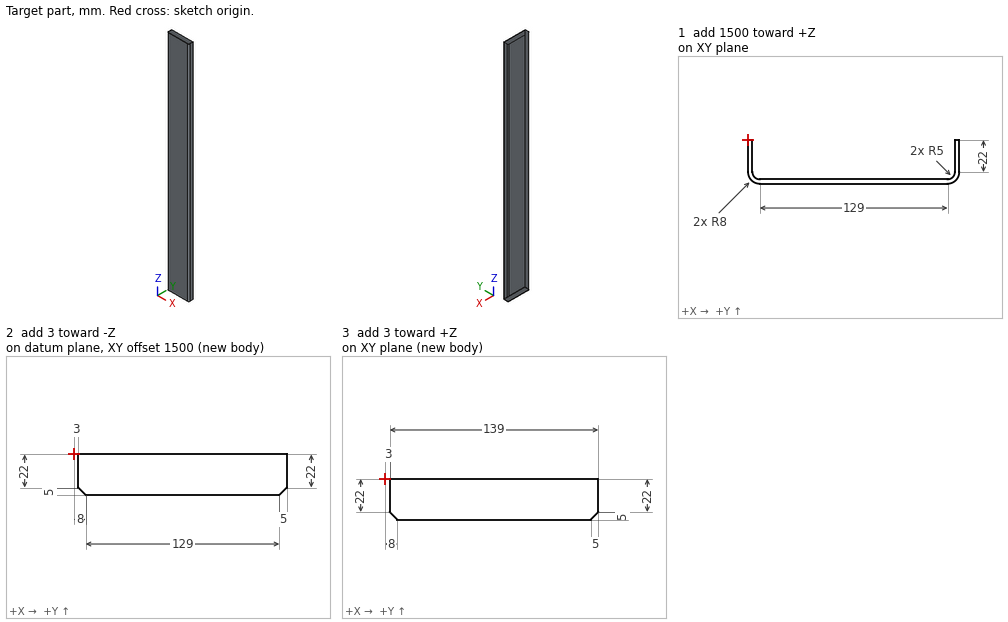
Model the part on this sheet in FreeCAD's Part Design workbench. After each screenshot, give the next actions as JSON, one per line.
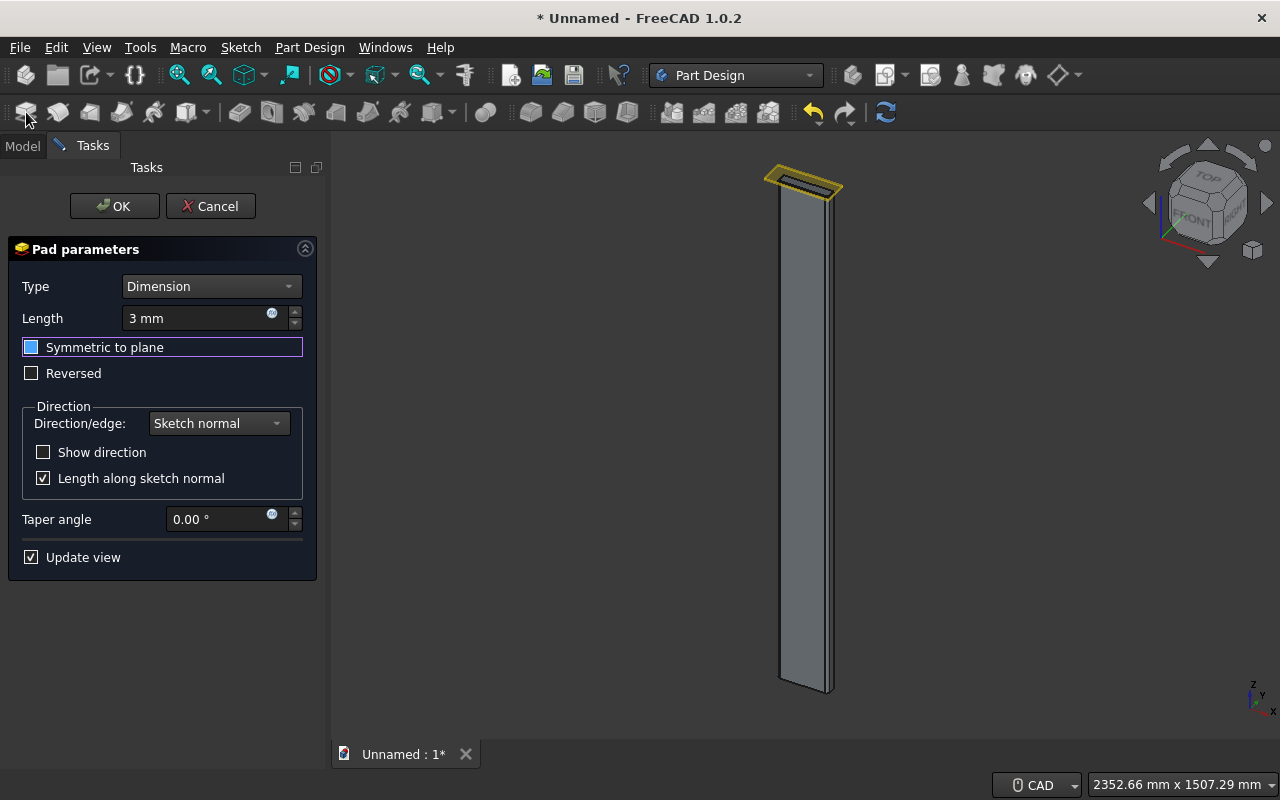
{"action": "left_click", "coordinate": [30, 373]}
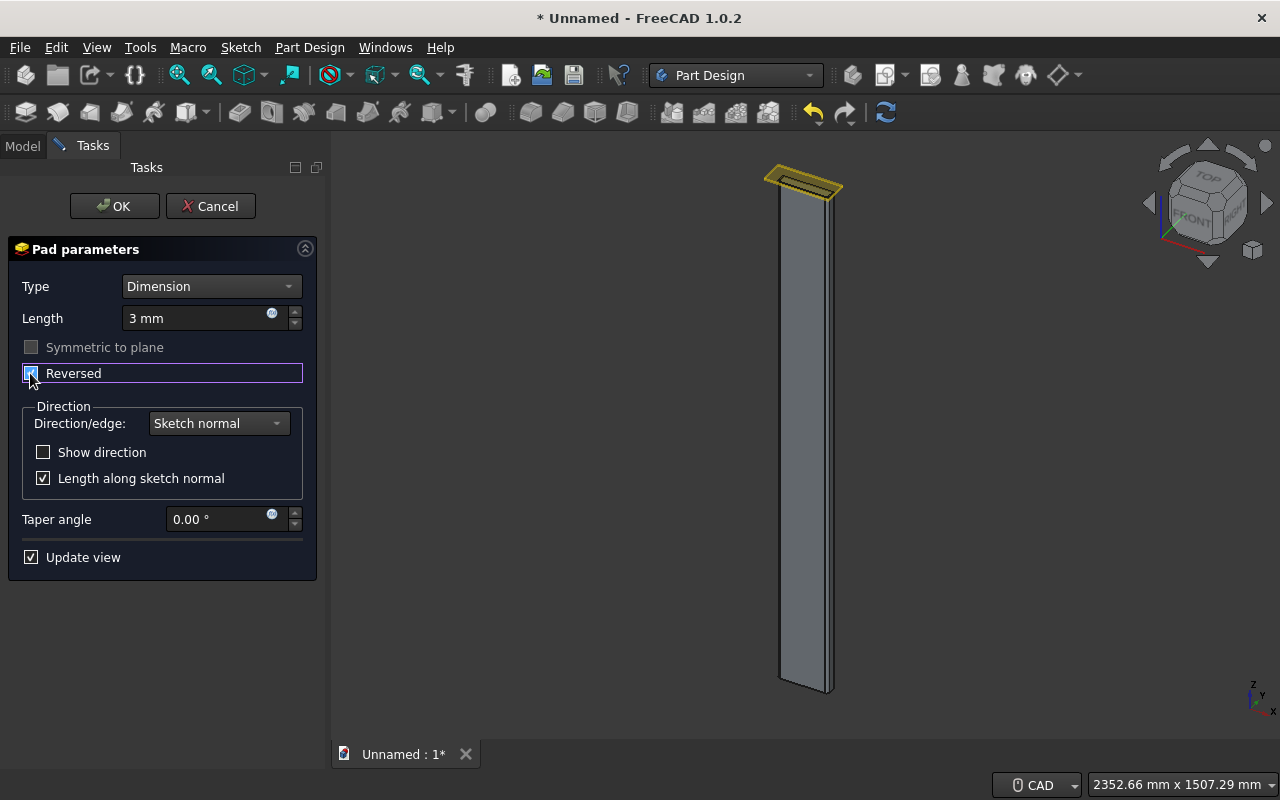
{"action": "left_click", "coordinate": [115, 206]}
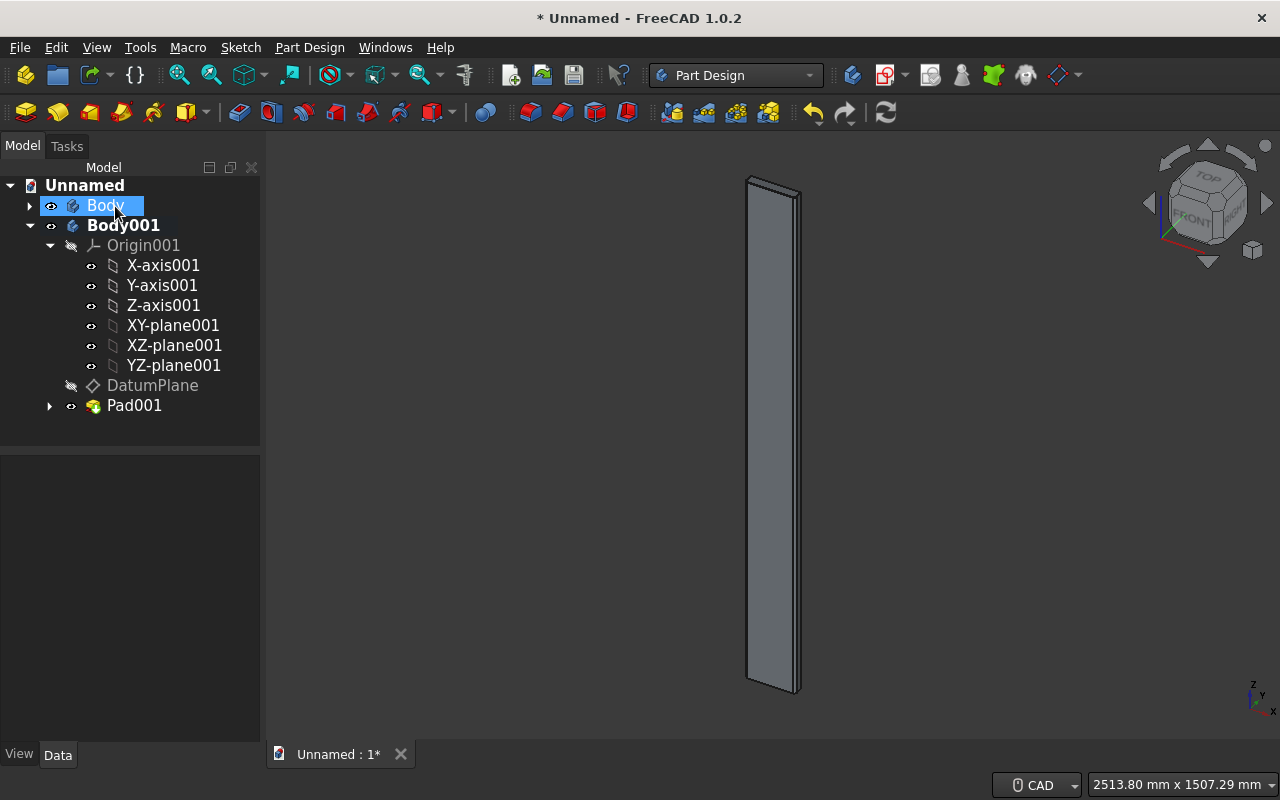
{"action": "key", "text": "v f"}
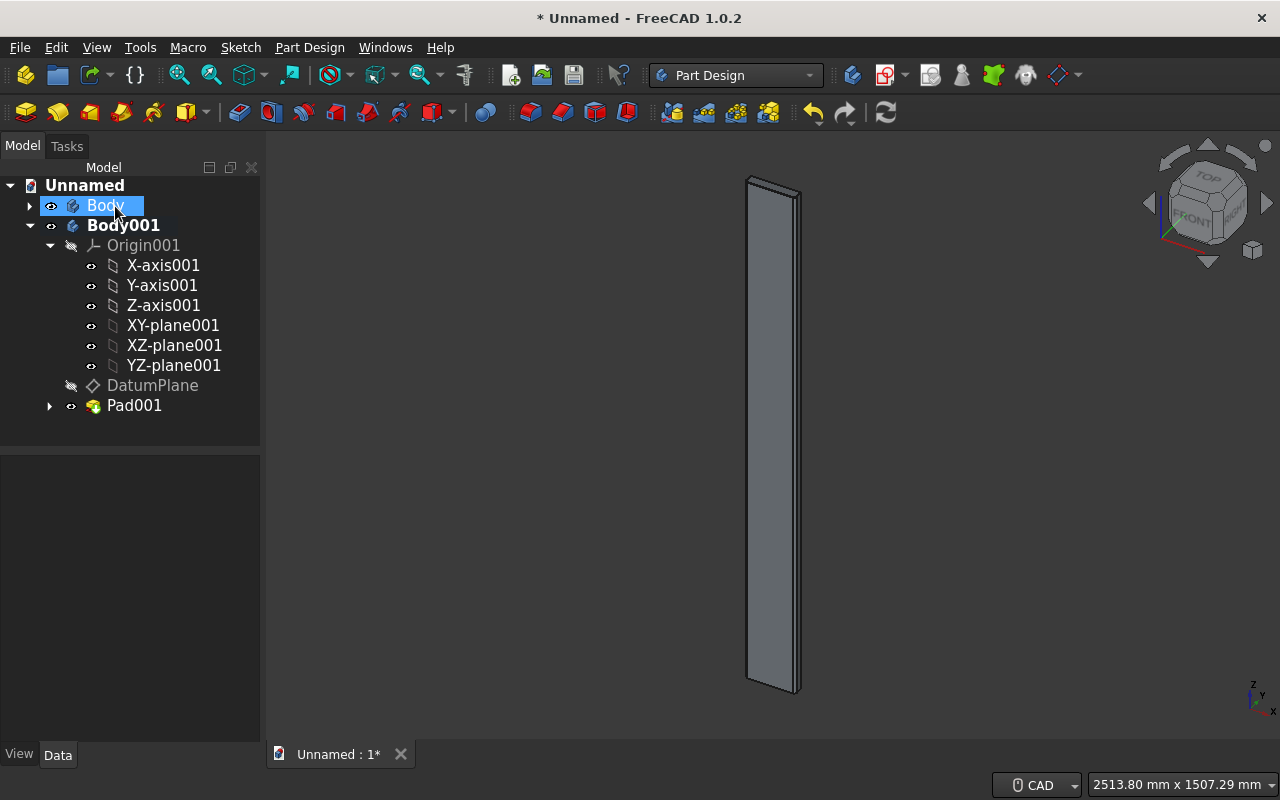
{"action": "left_click", "coordinate": [854, 76]}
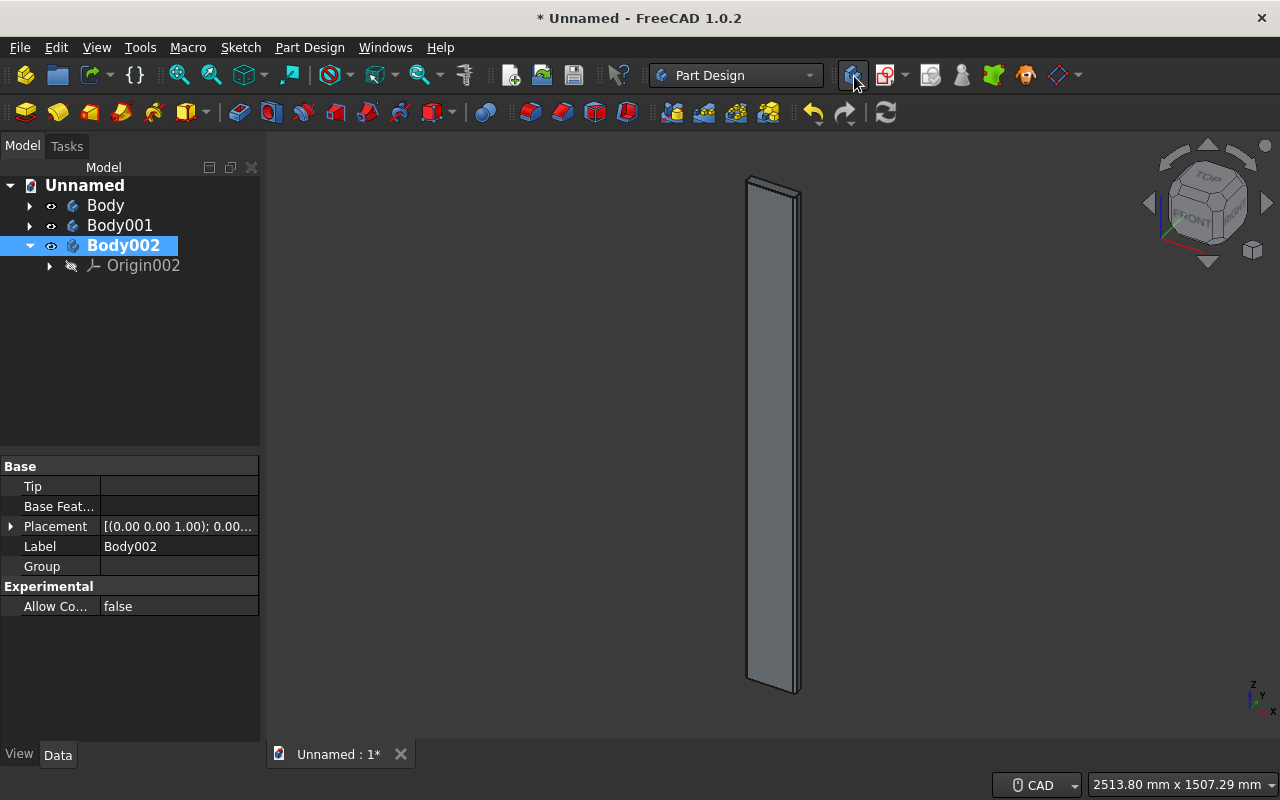
{"action": "left_click", "coordinate": [306, 699]}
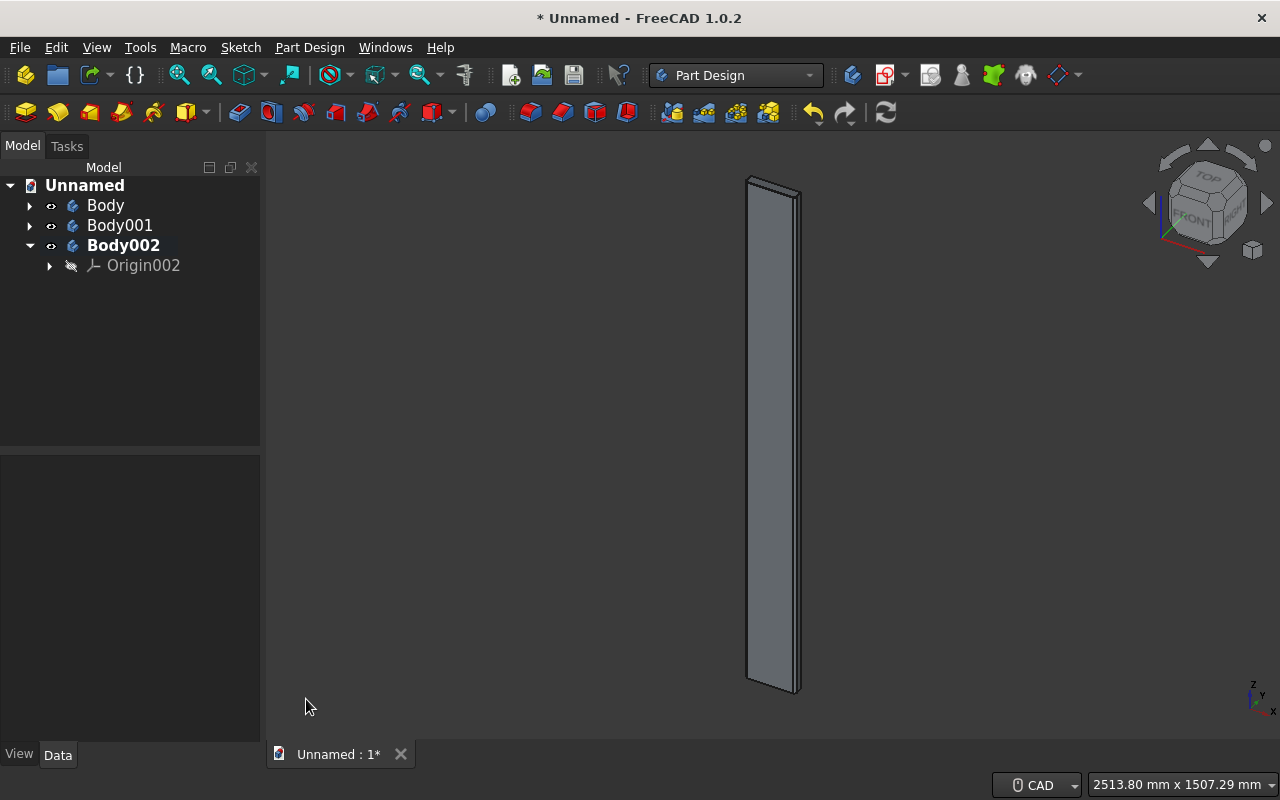
{"action": "left_click", "coordinate": [886, 76]}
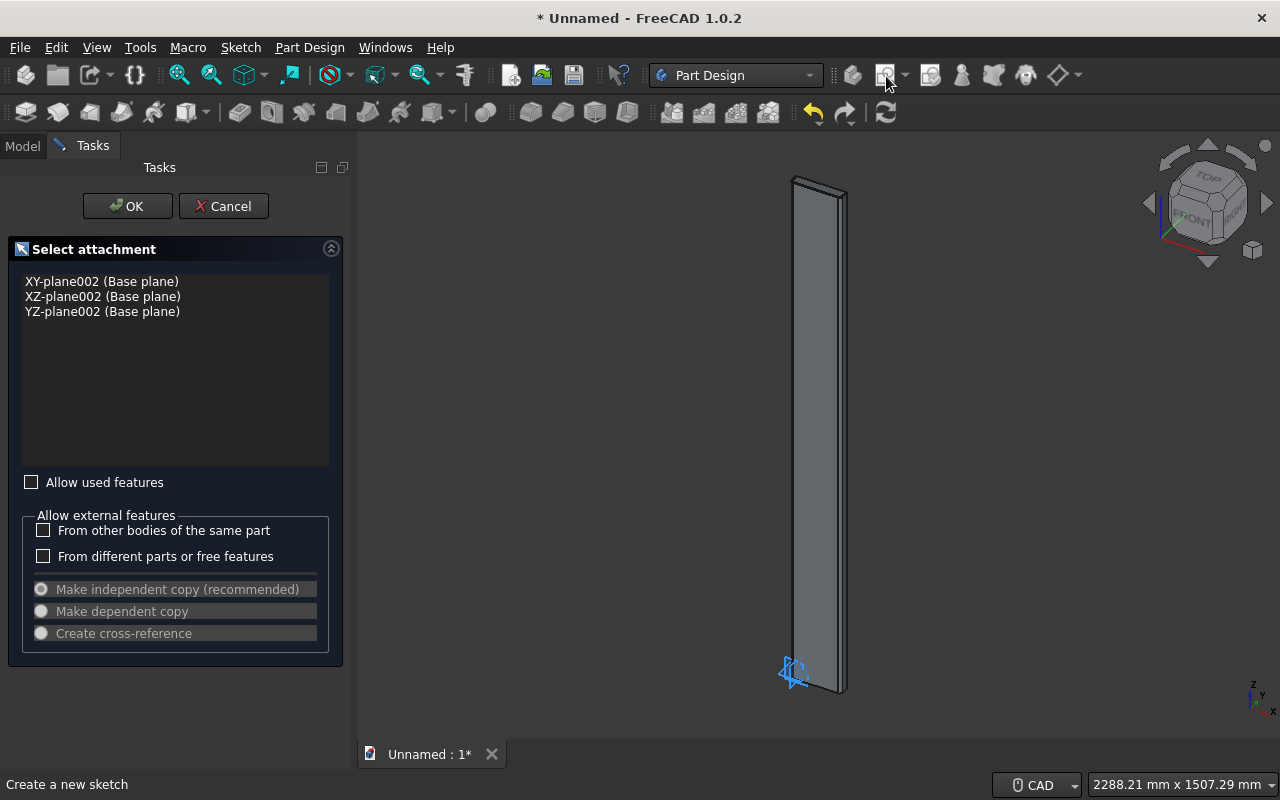
{"action": "left_click", "coordinate": [82, 282]}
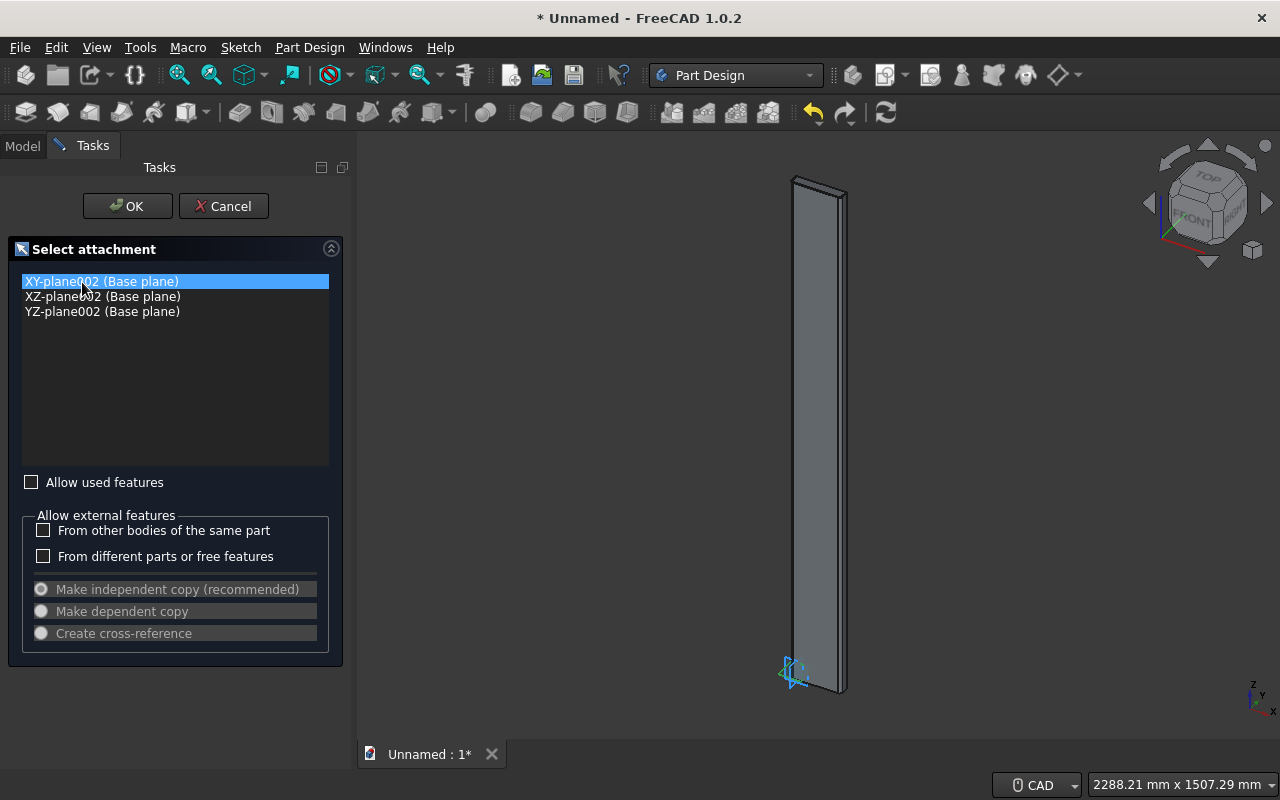
{"action": "left_click", "coordinate": [128, 206]}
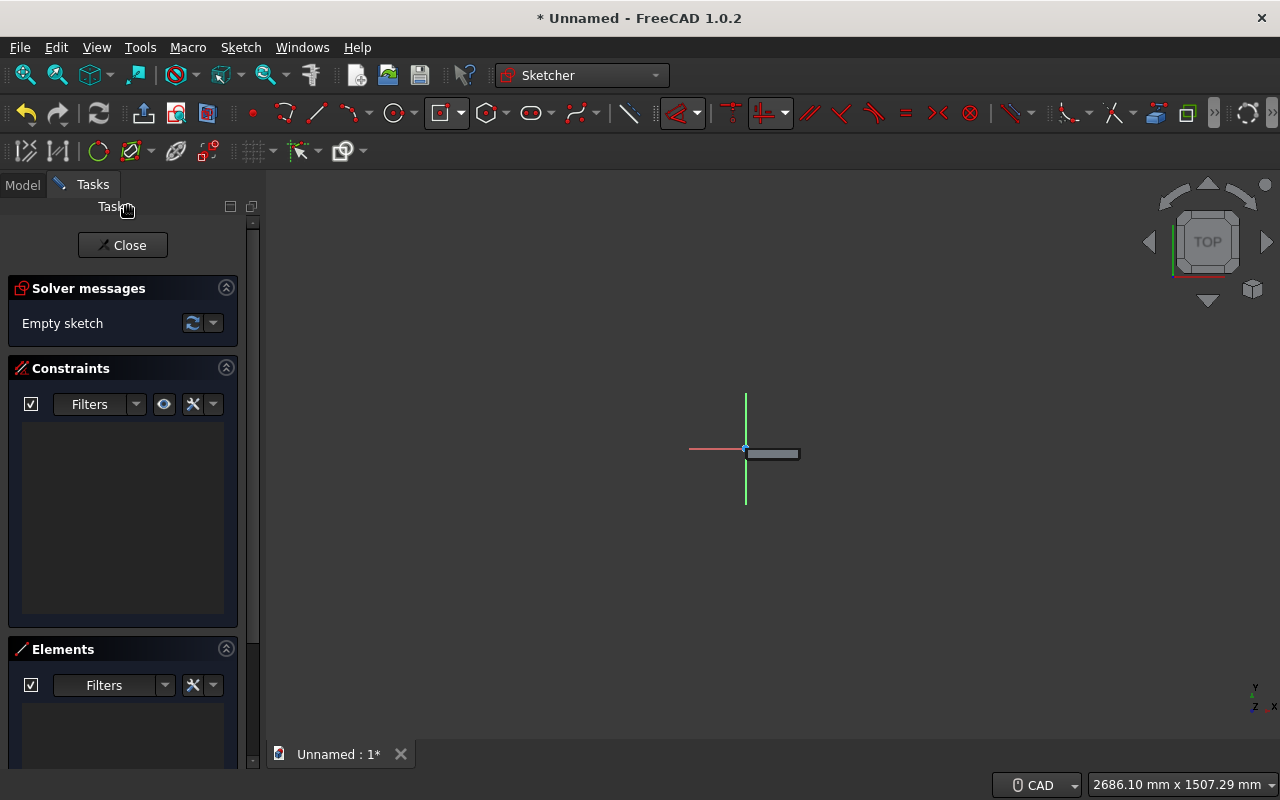
{"action": "scroll", "coordinate": [779, 454], "scroll_direction": "up", "scroll_amount": 12}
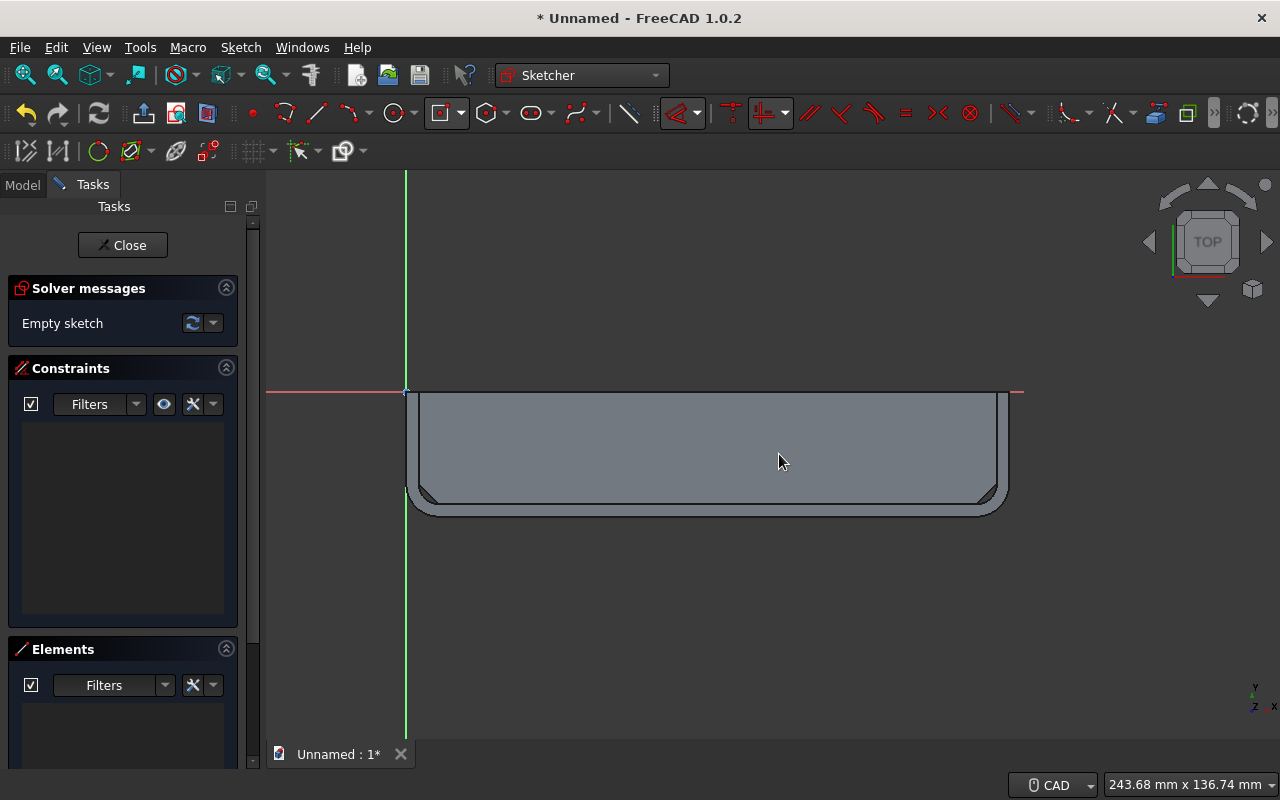
{"action": "key", "text": "g m"}